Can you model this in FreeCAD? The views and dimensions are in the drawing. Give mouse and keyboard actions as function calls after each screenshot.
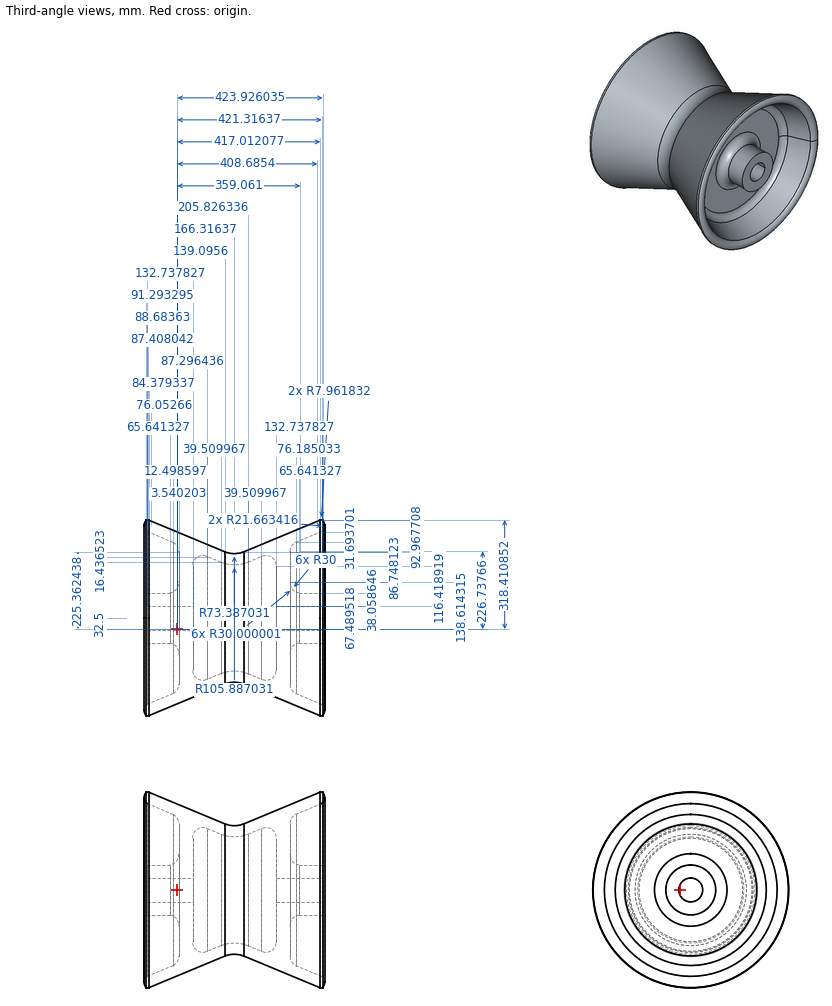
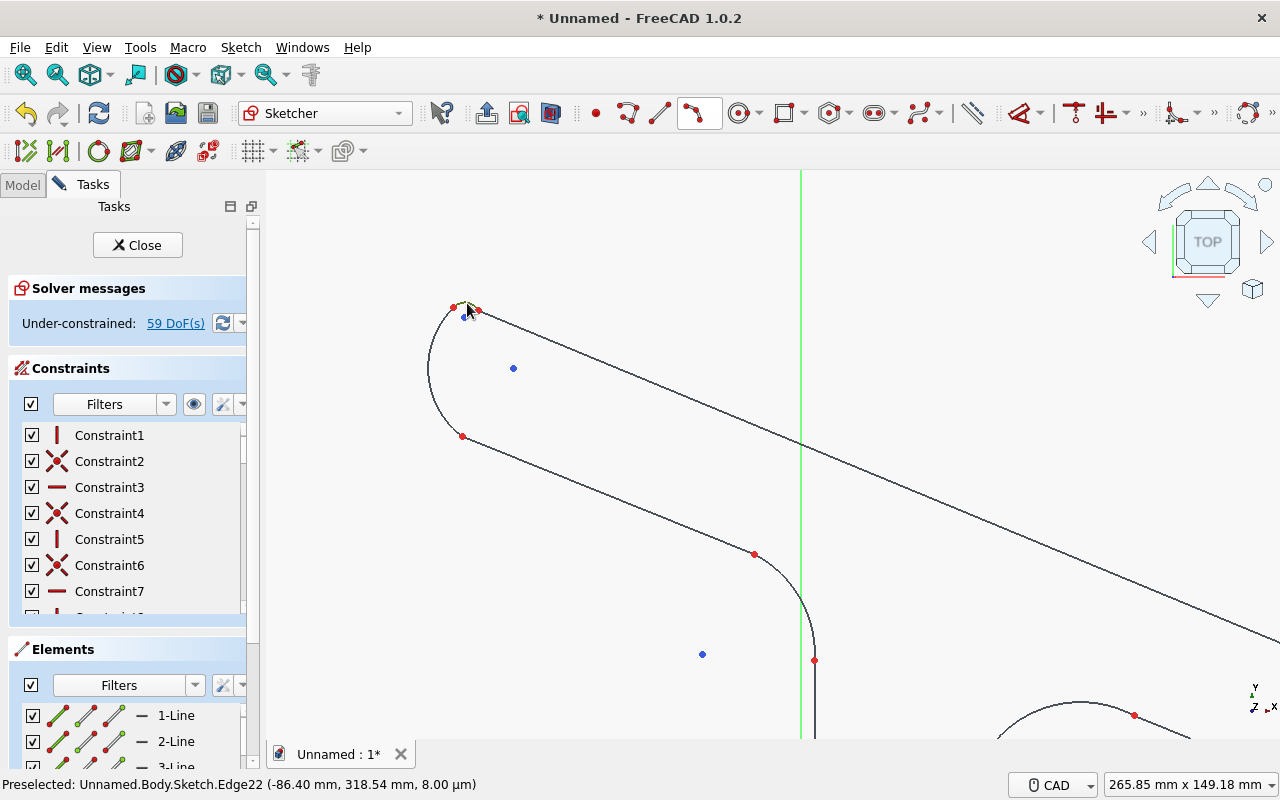
key(e)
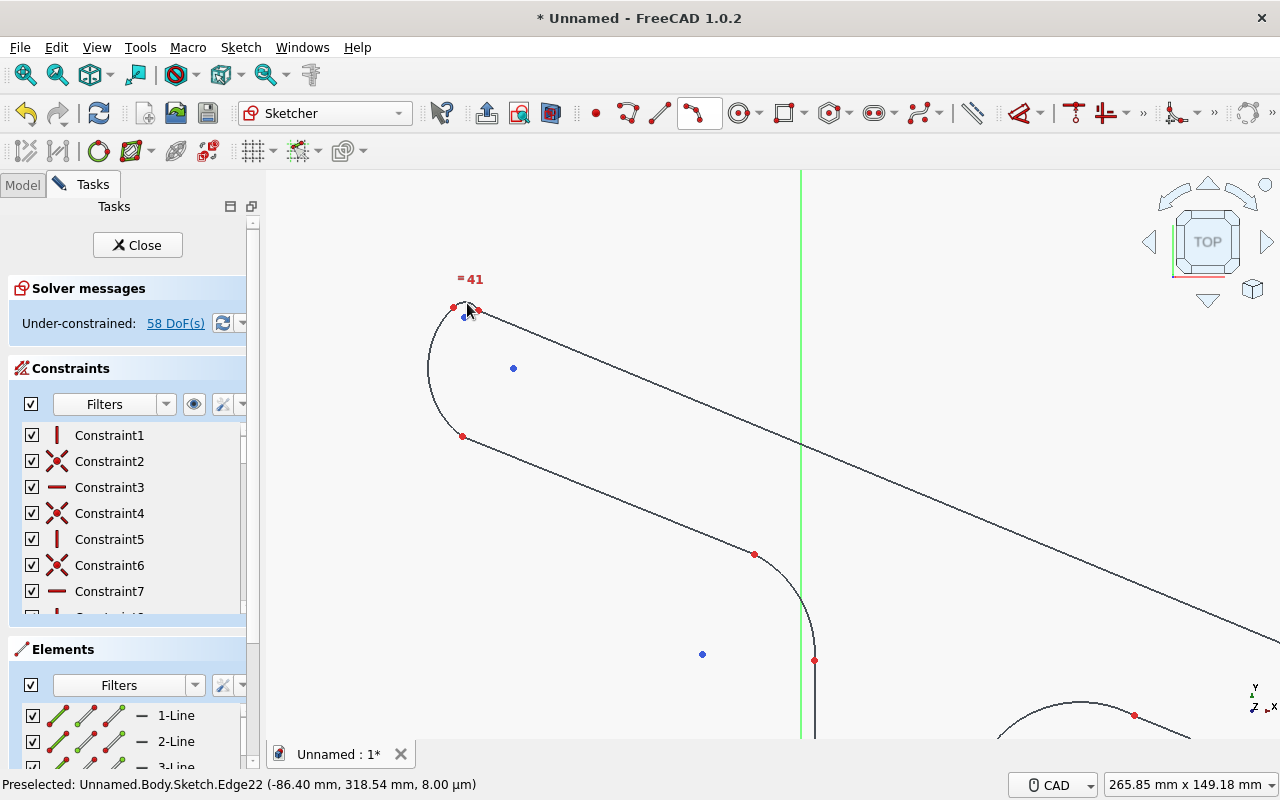
scroll(465, 305, down, 7)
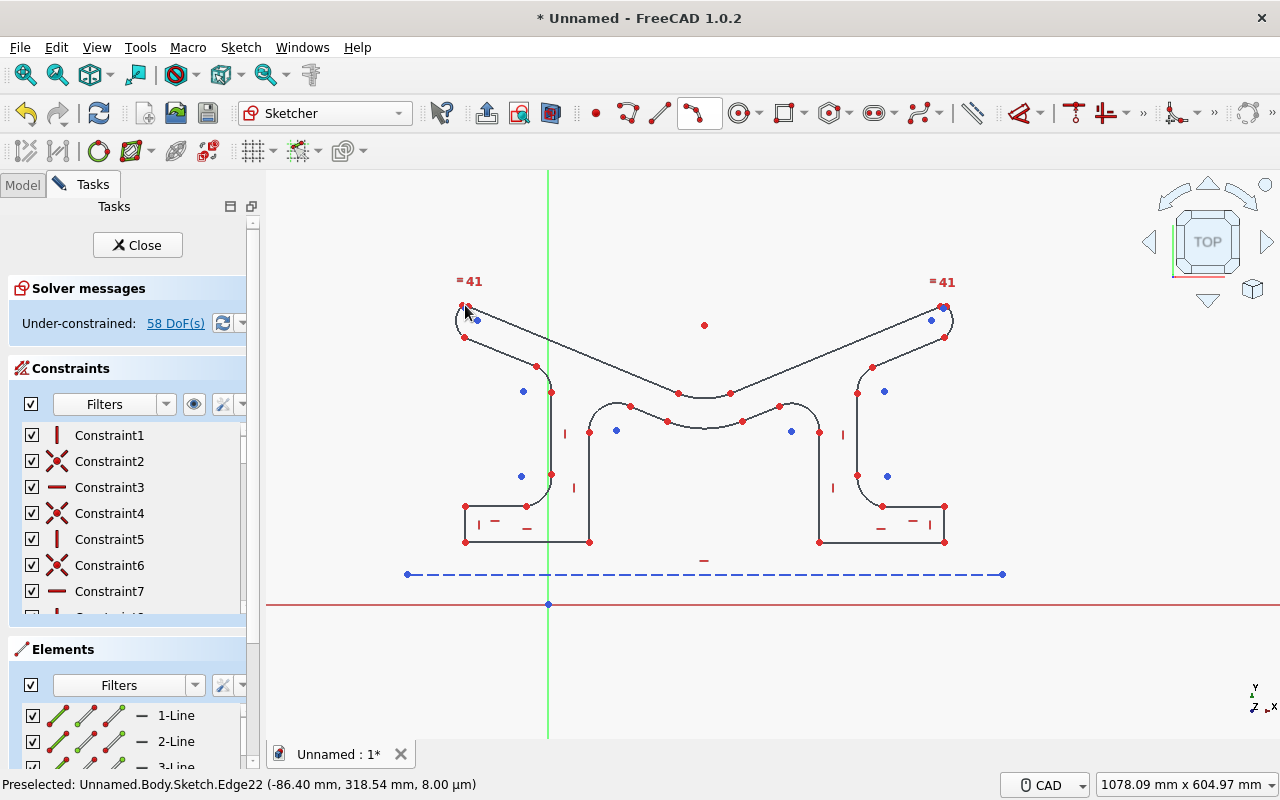
scroll(951, 329, up, 2)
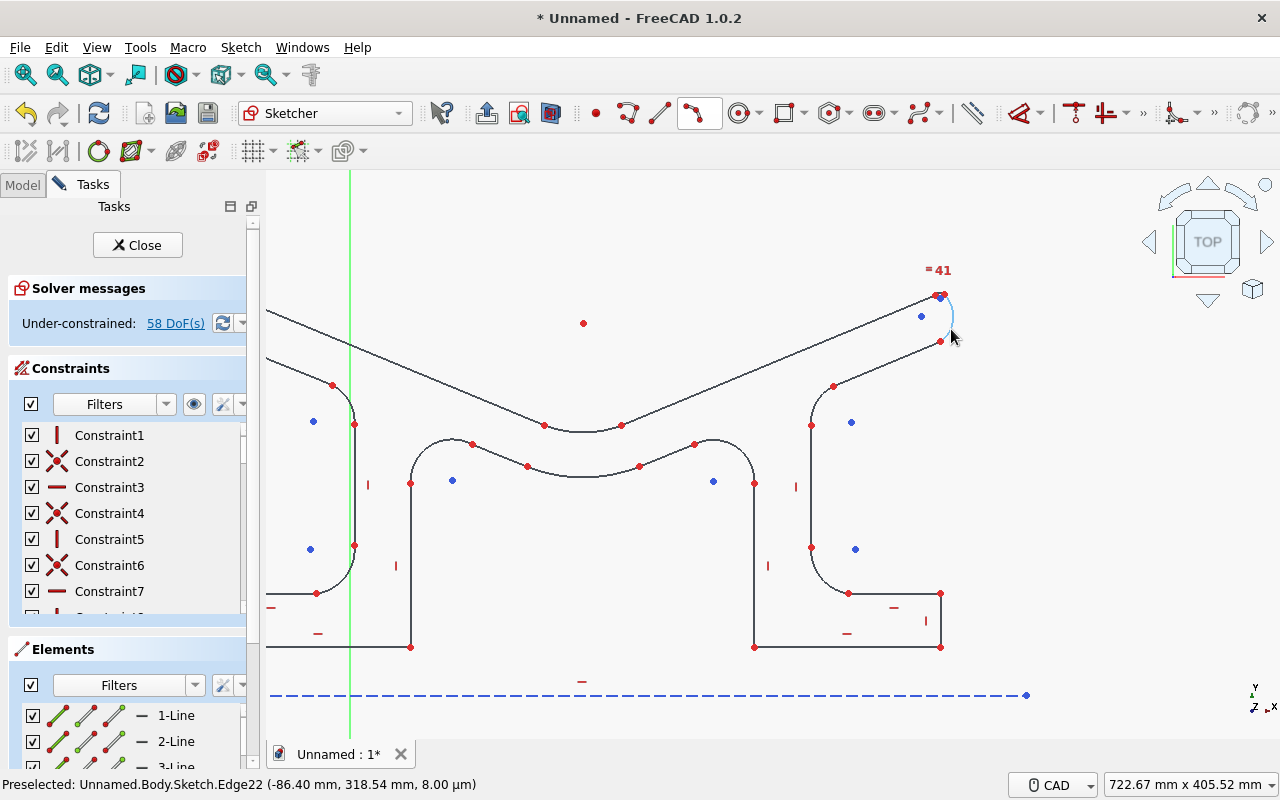
click(951, 329)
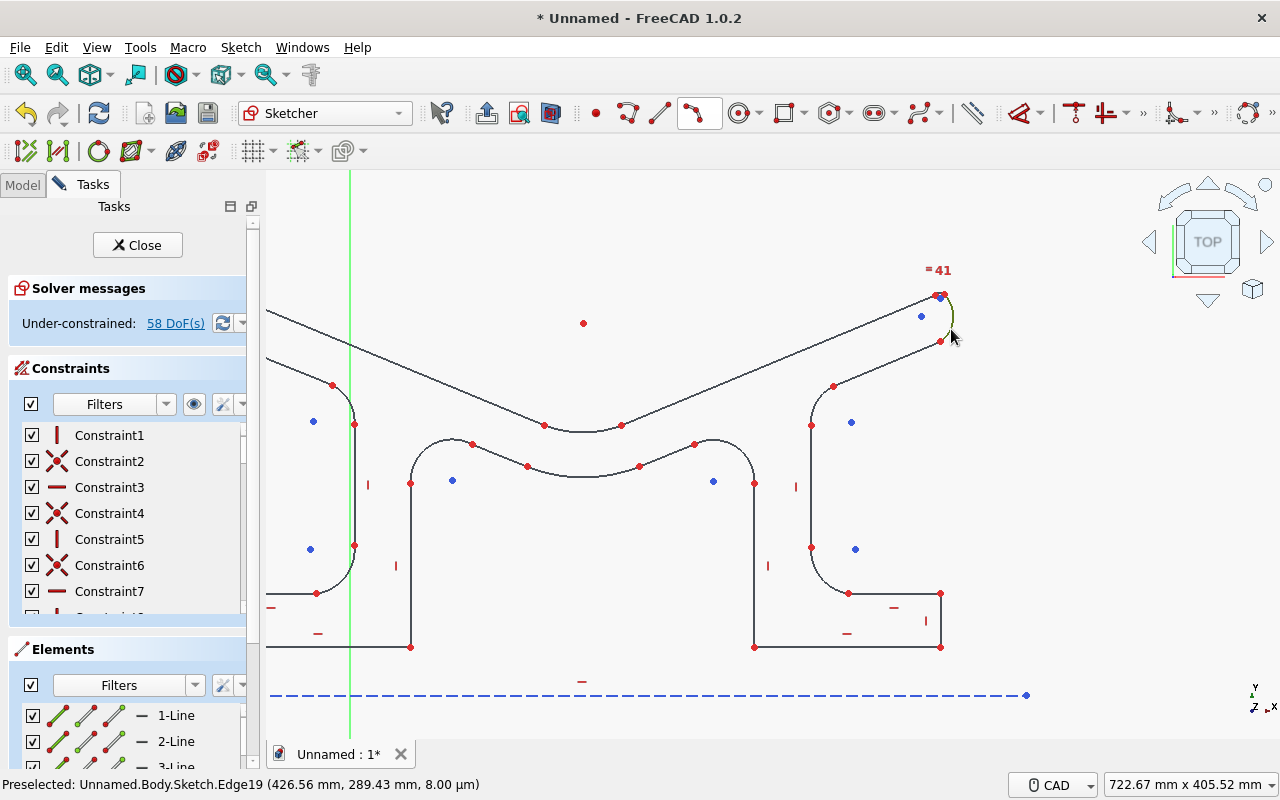
scroll(952, 329, down, 2)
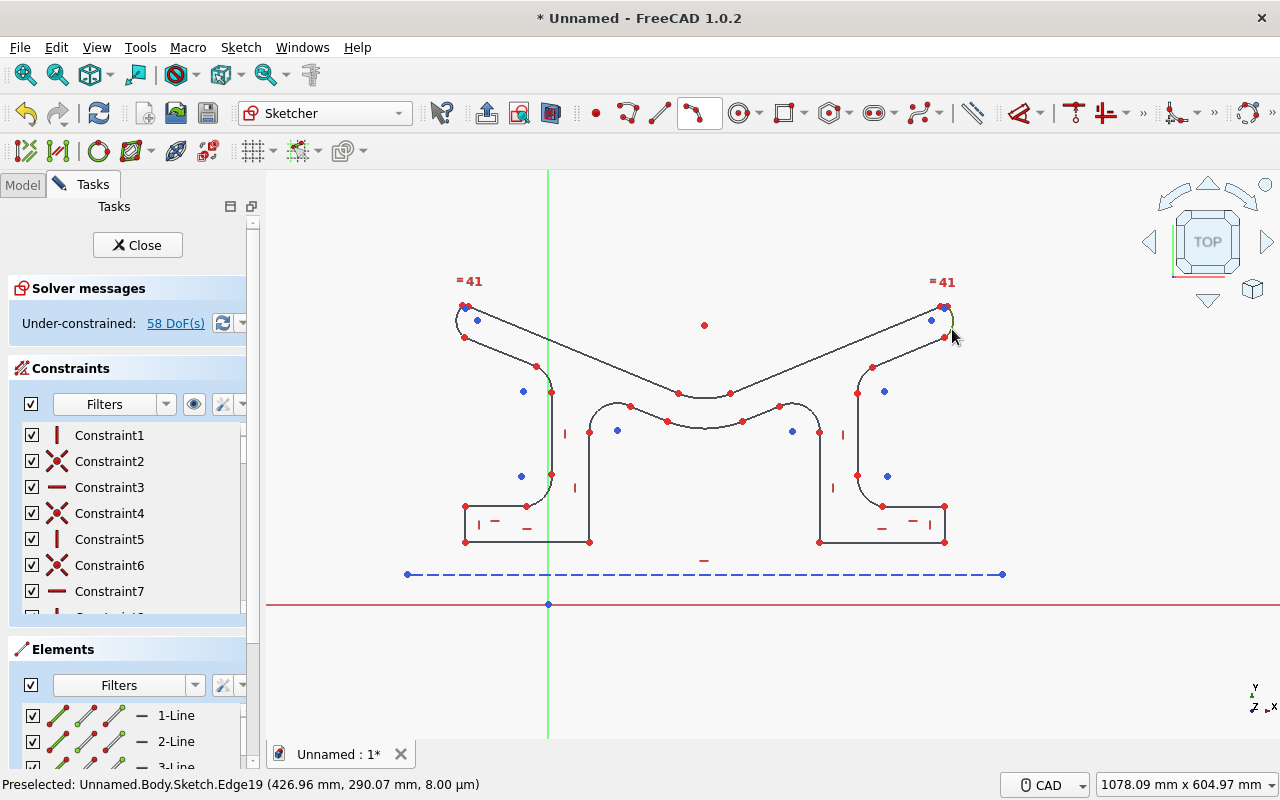
scroll(457, 315, up, 2)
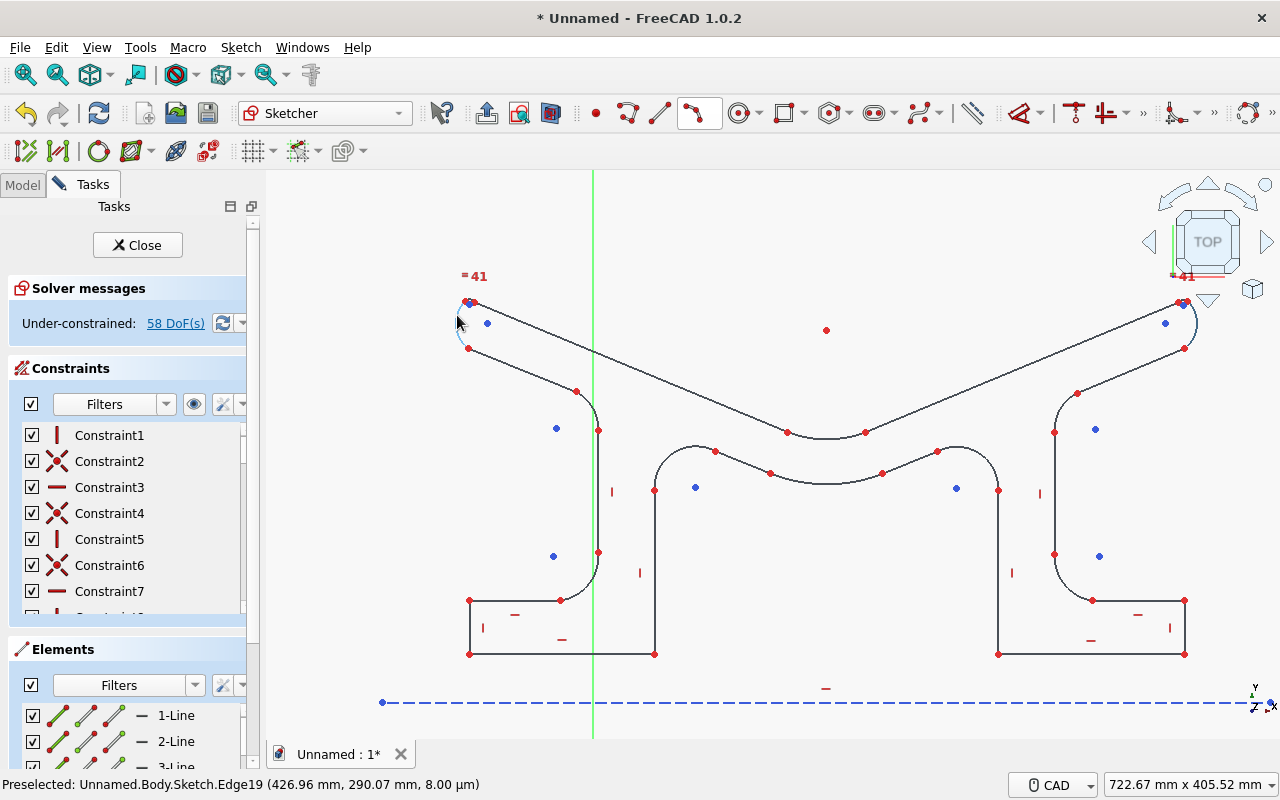
click(457, 315)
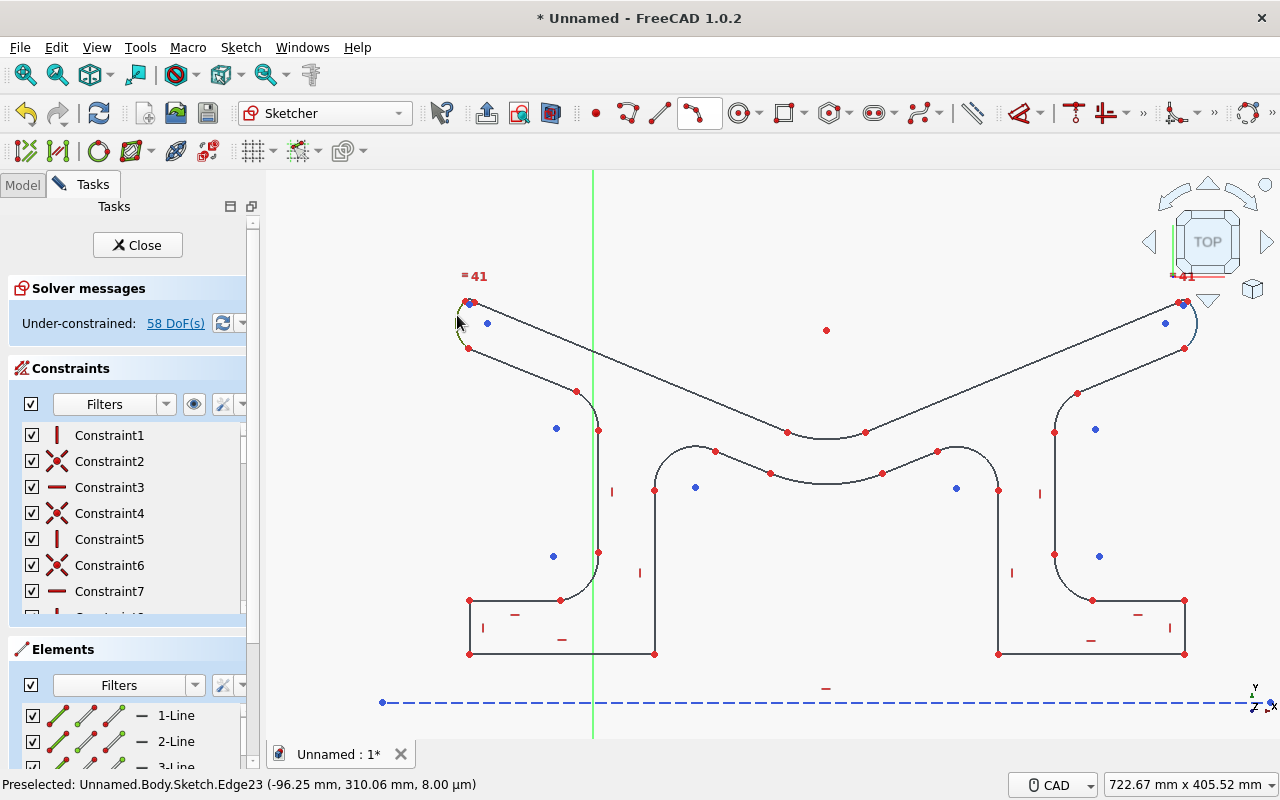
key(e)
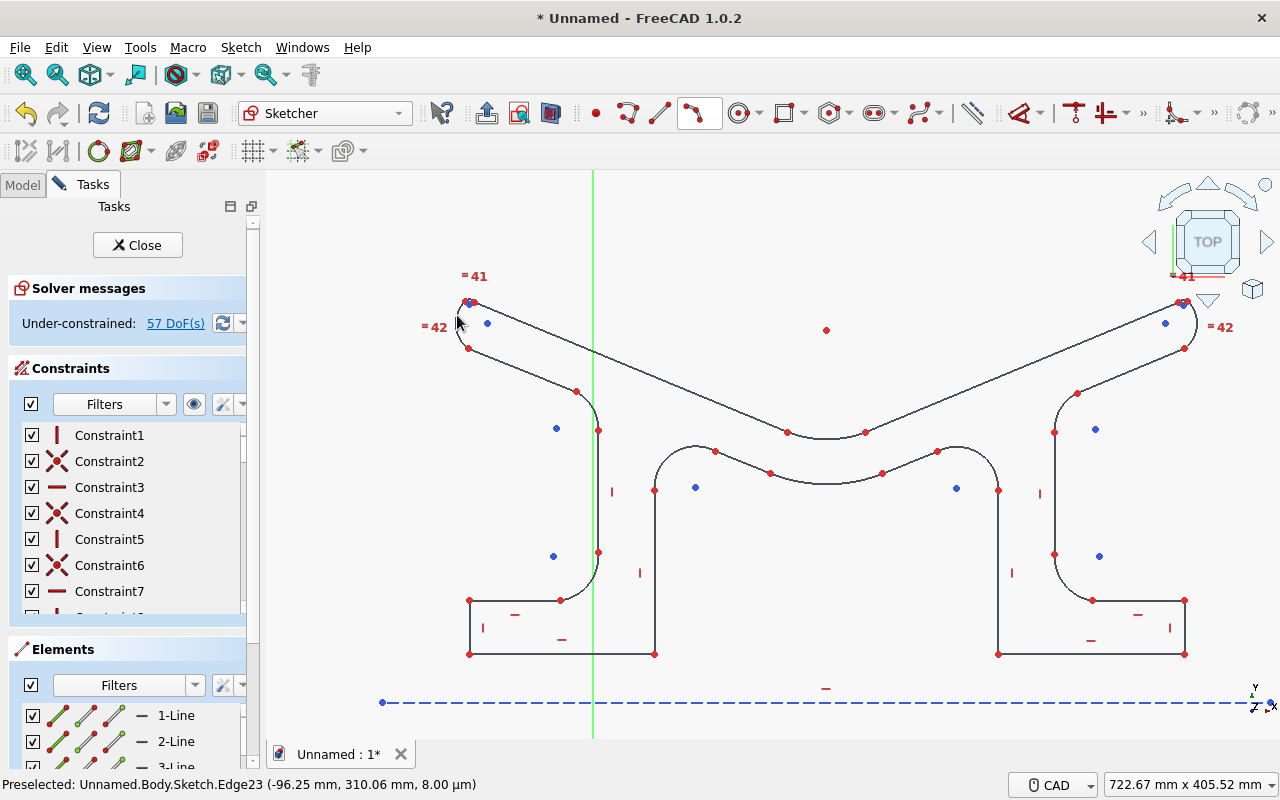
click(1058, 573)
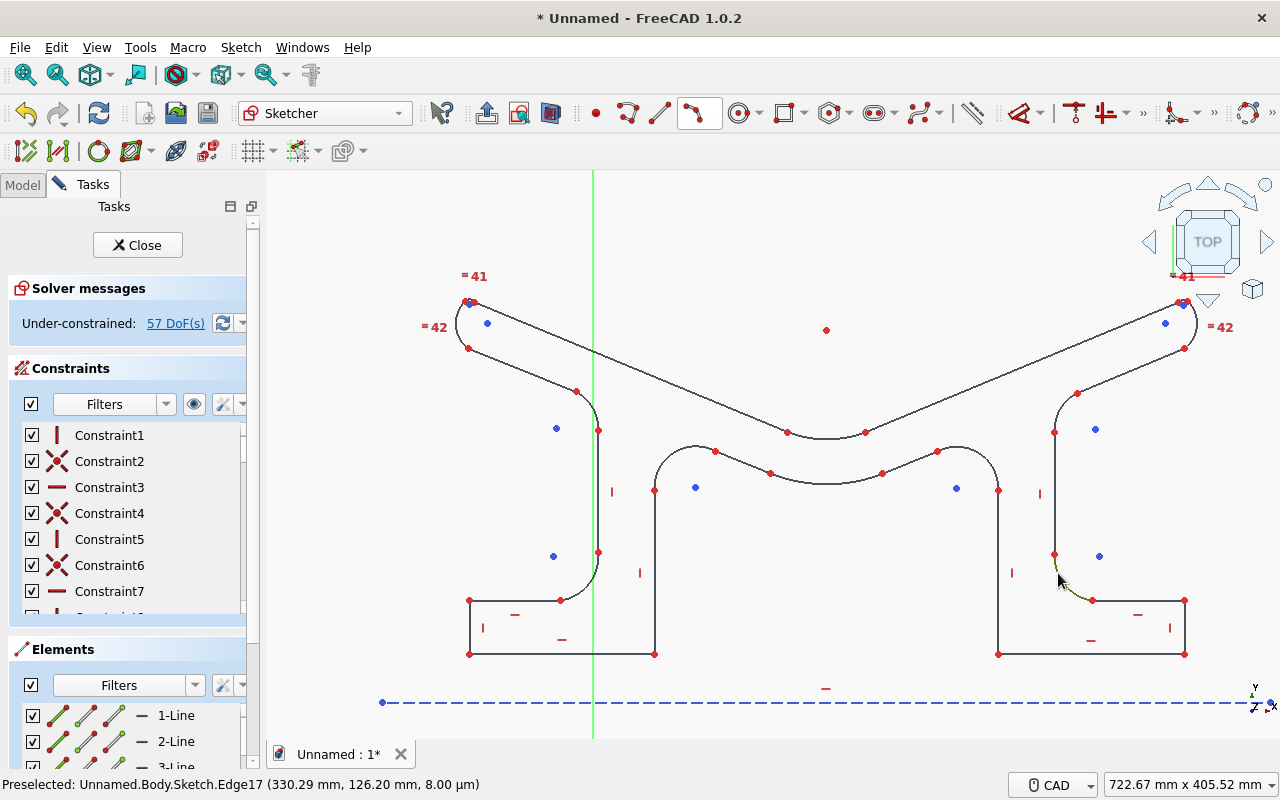
click(597, 417)